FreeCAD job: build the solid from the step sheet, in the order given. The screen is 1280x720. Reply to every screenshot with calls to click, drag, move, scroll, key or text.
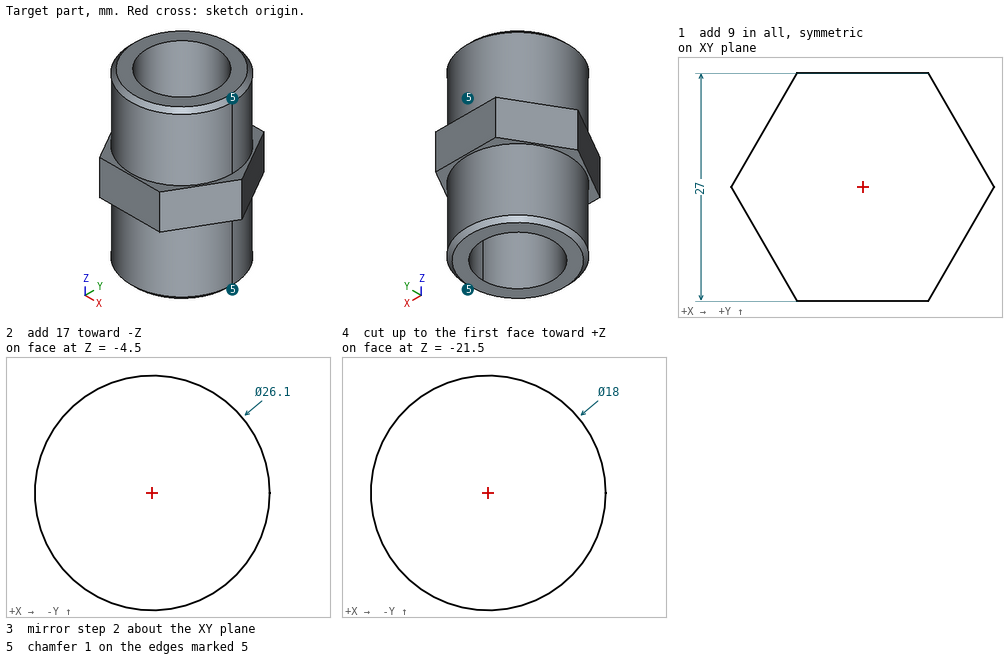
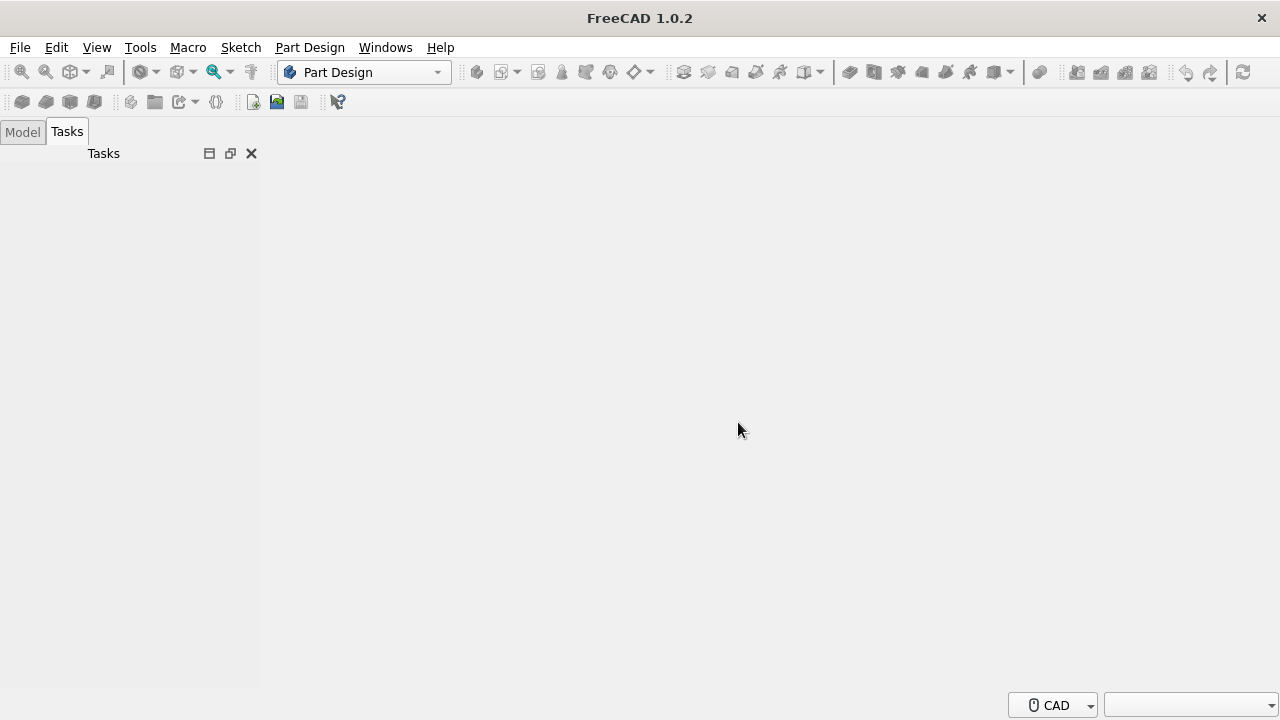
click(254, 102)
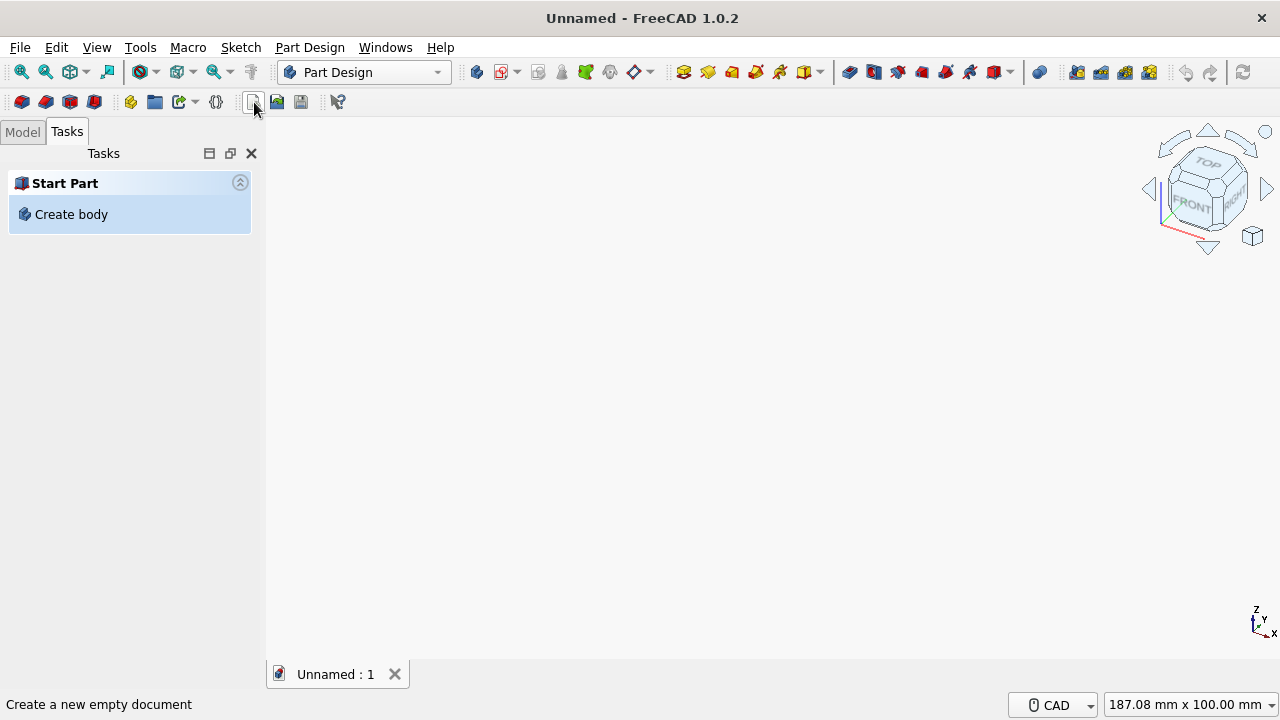
click(502, 72)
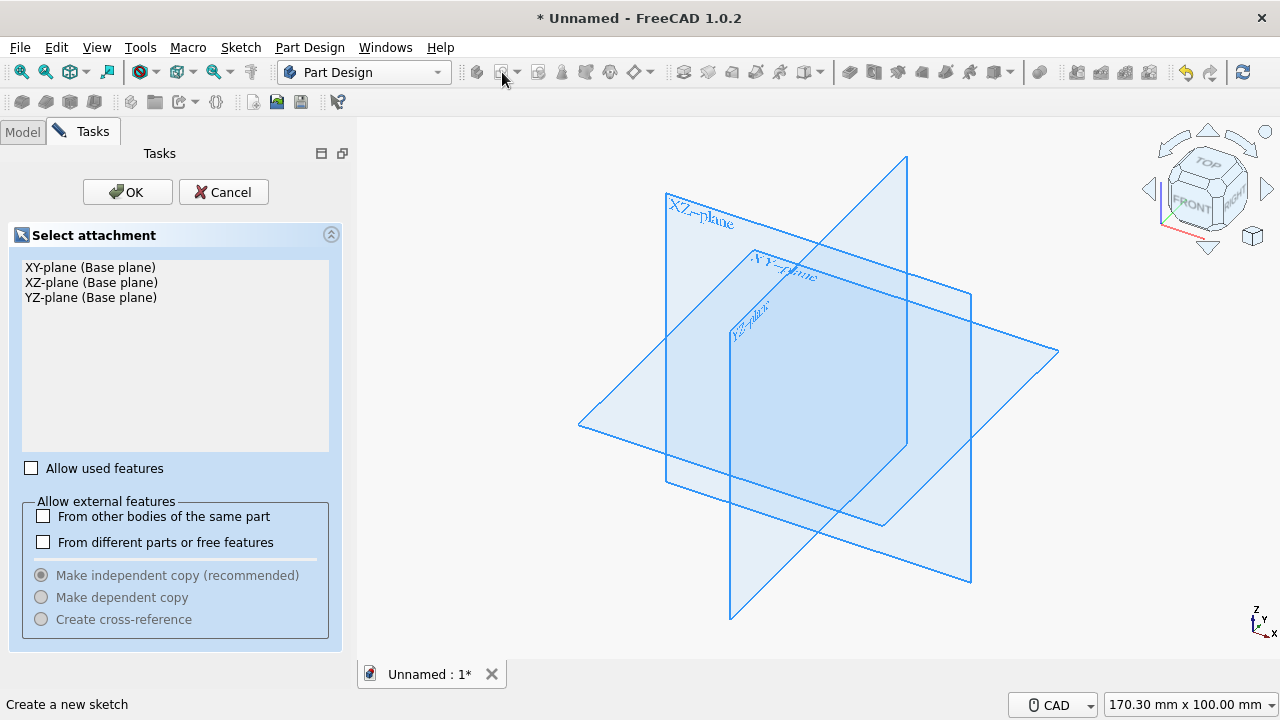
click(82, 268)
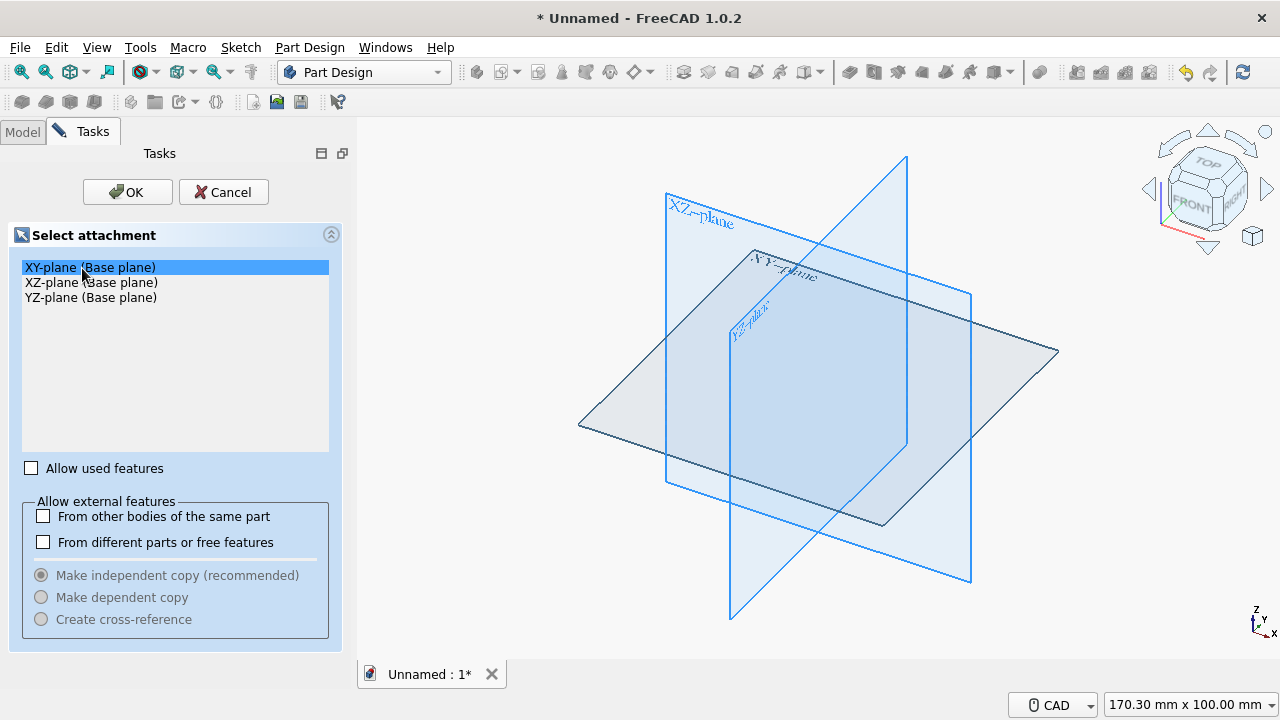
click(128, 192)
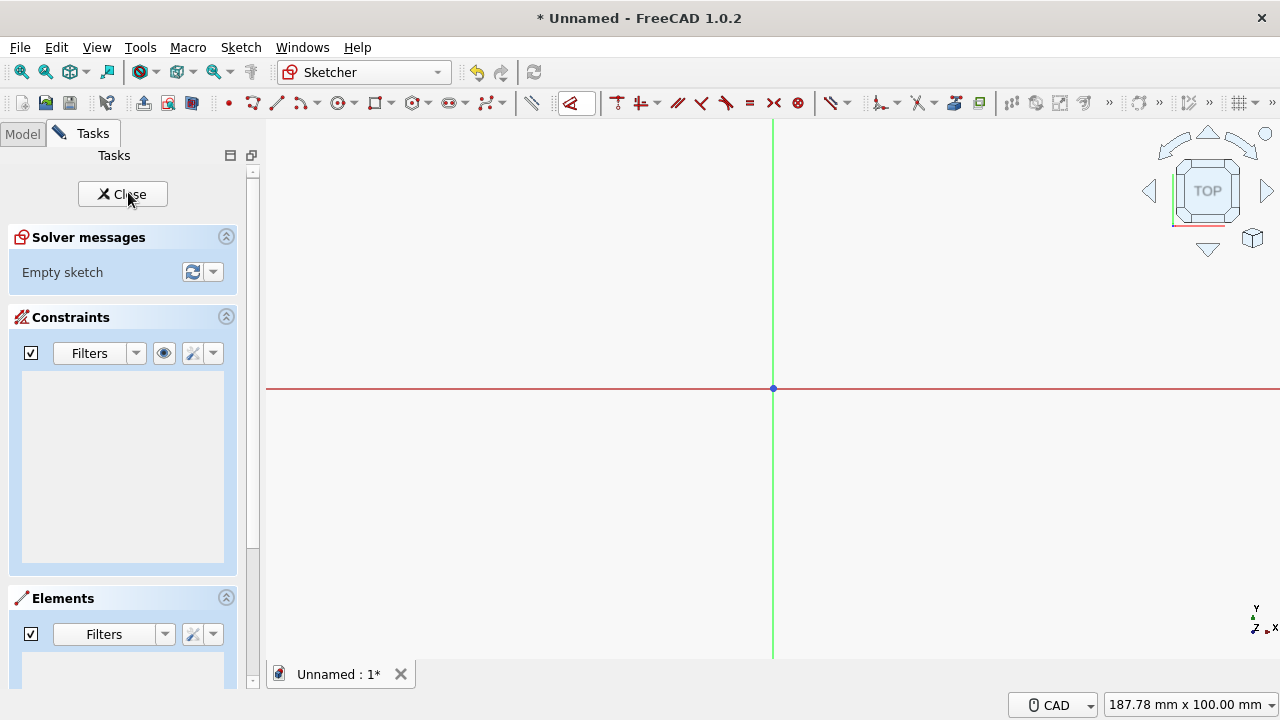
scroll(829, 389, up, 4)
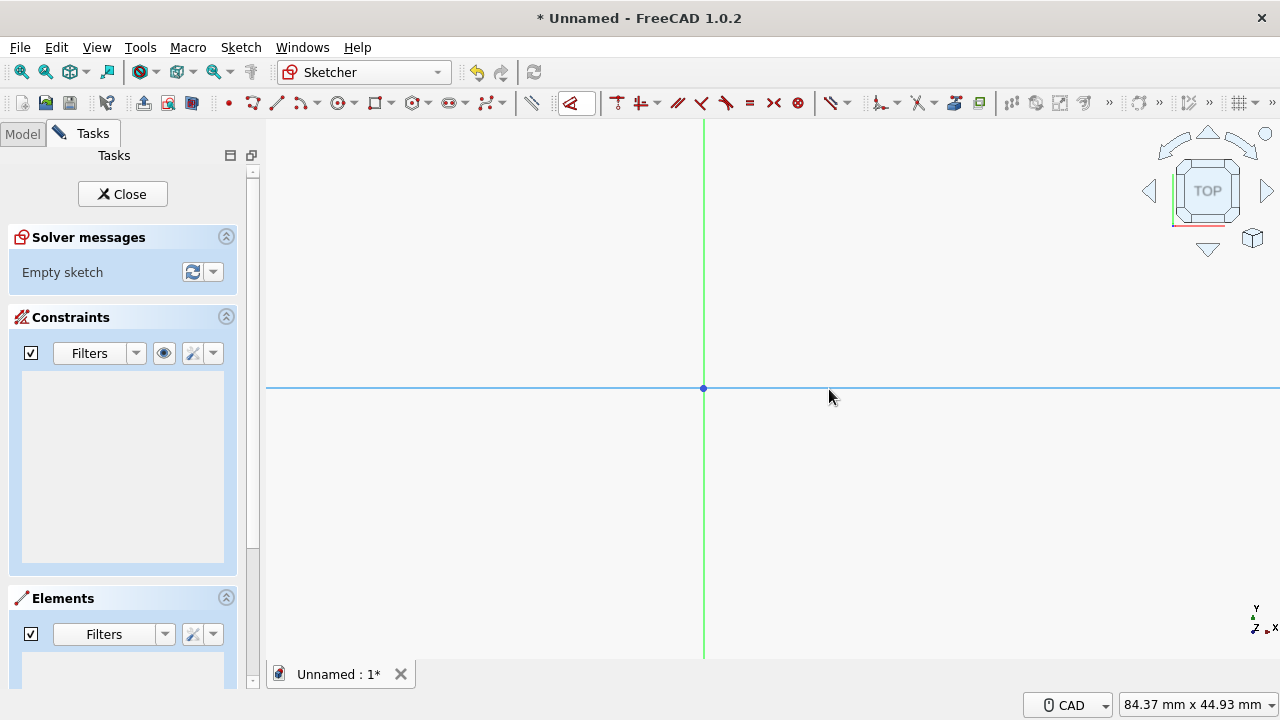
click(412, 104)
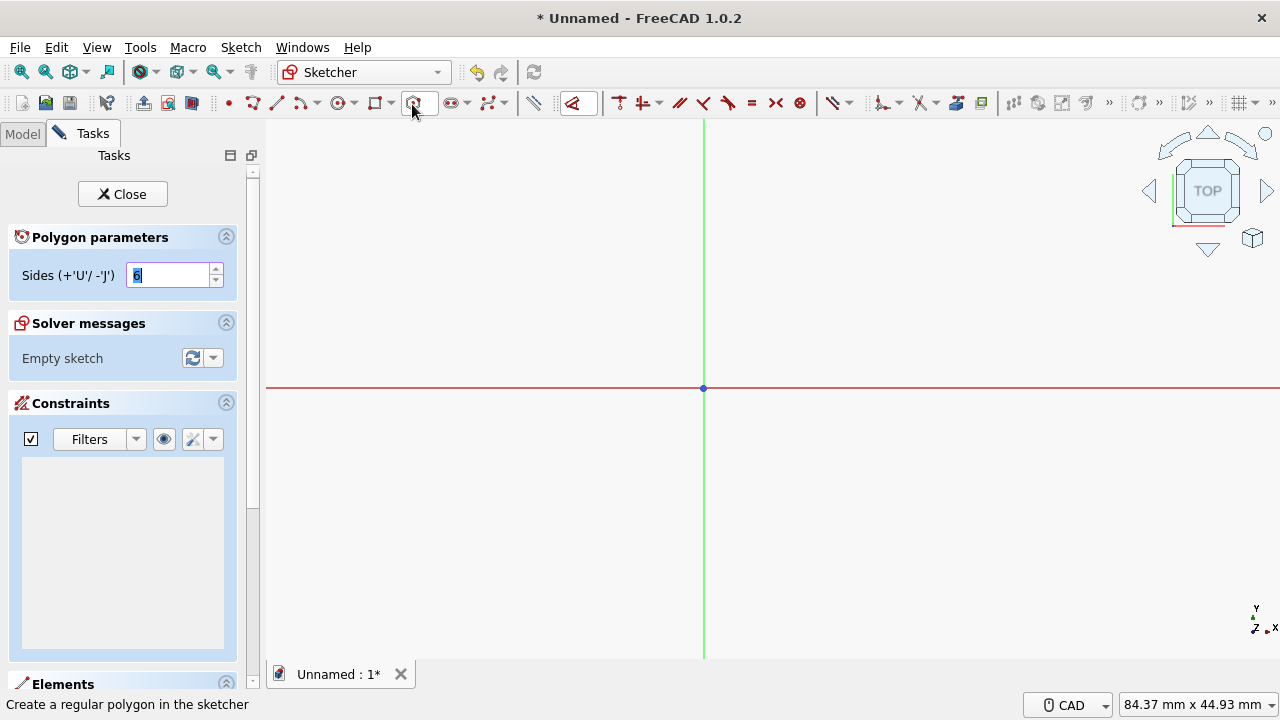
click(704, 388)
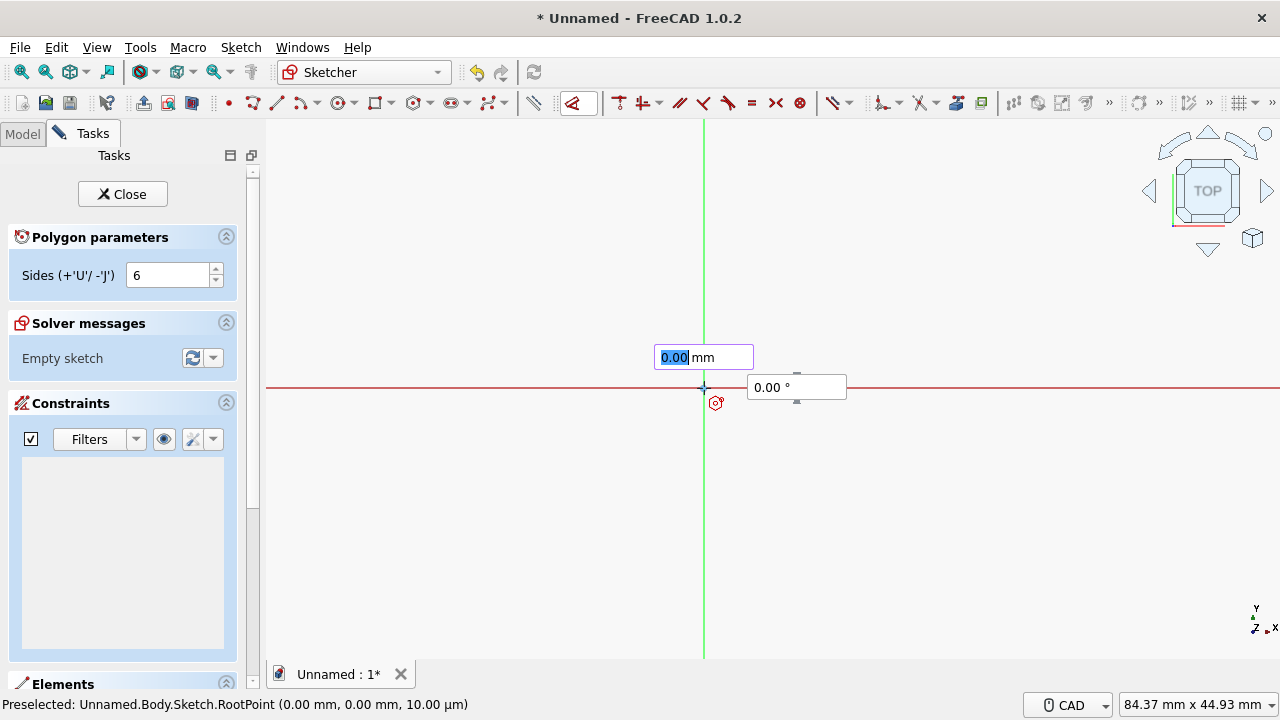
click(891, 388)
right_click(891, 388)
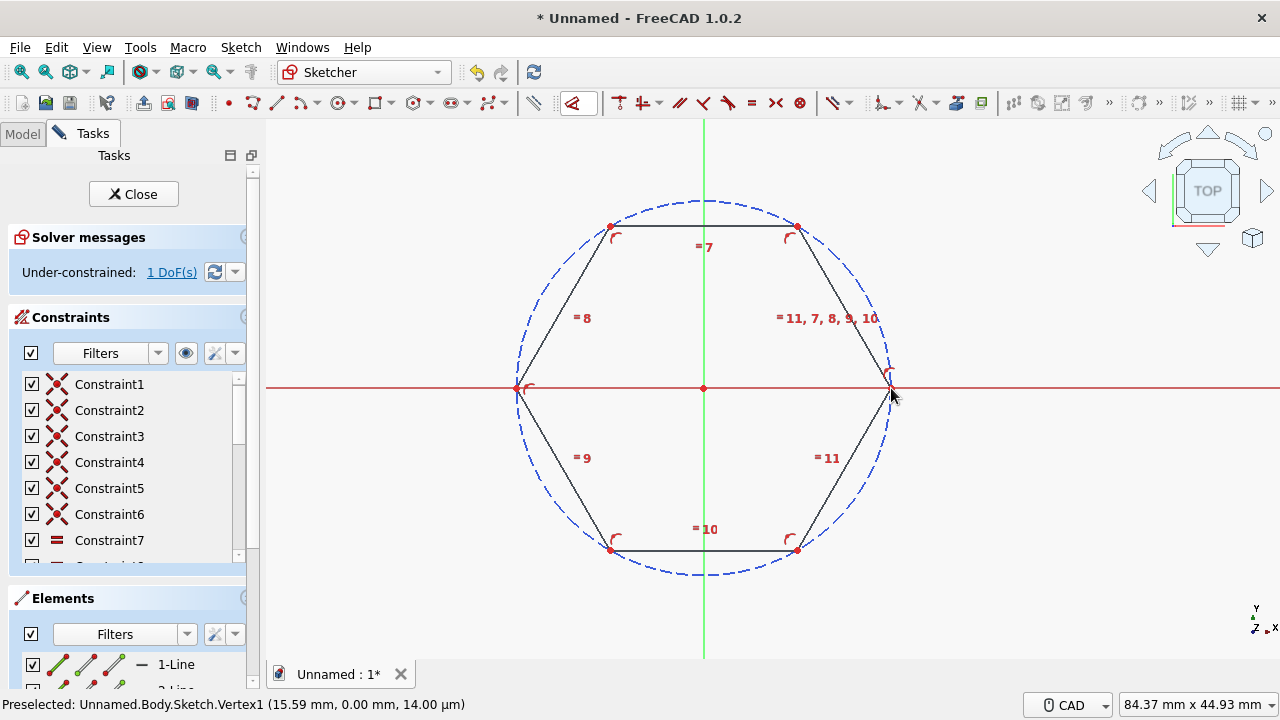
key(d)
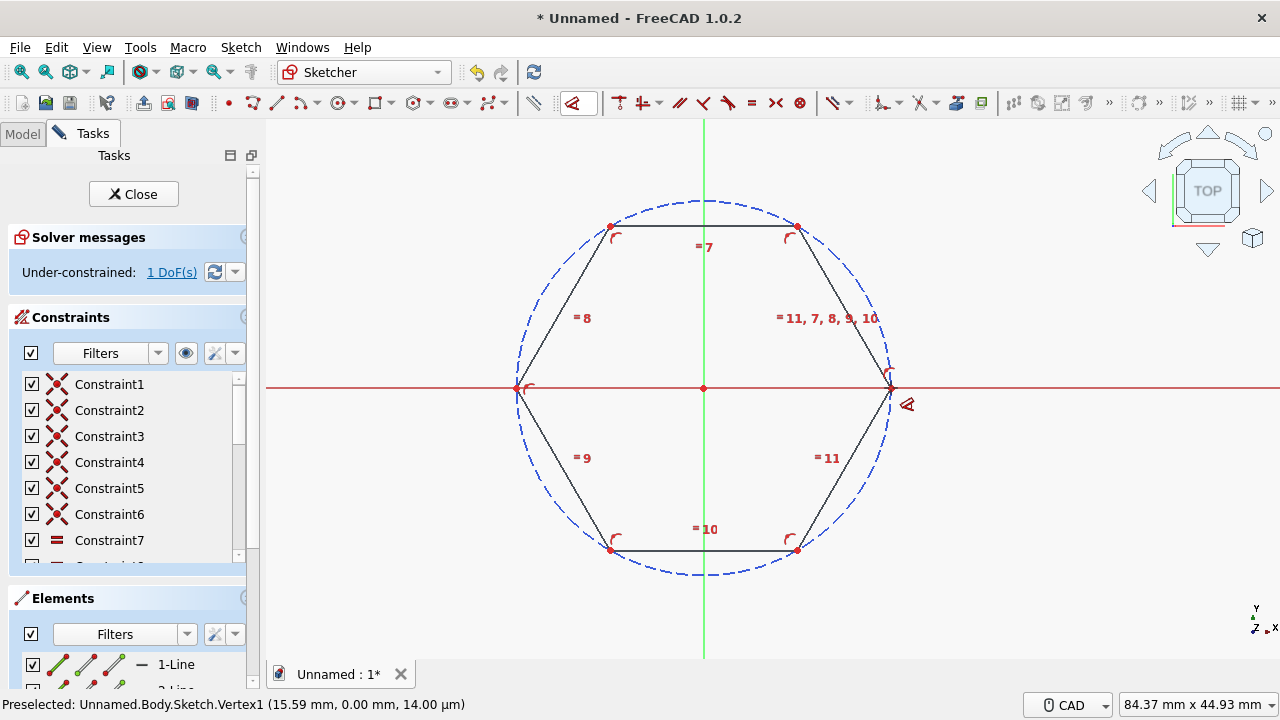
click(610, 551)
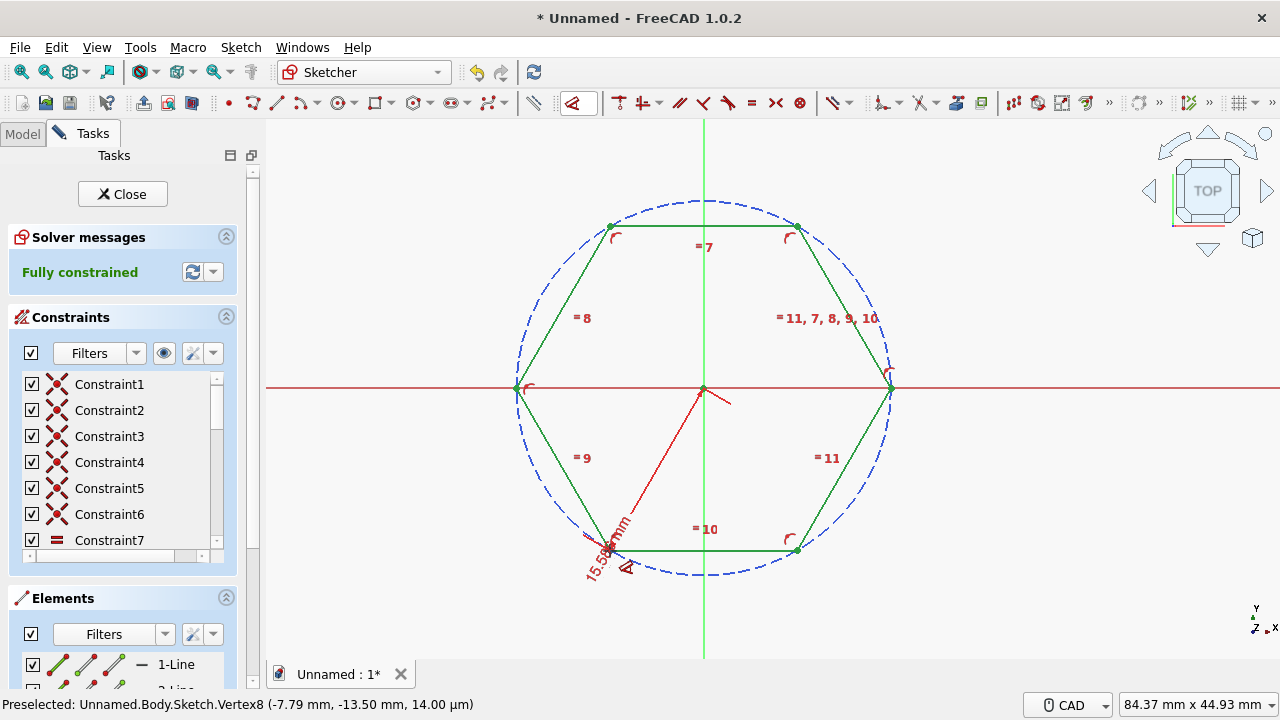
click(797, 226)
click(831, 314)